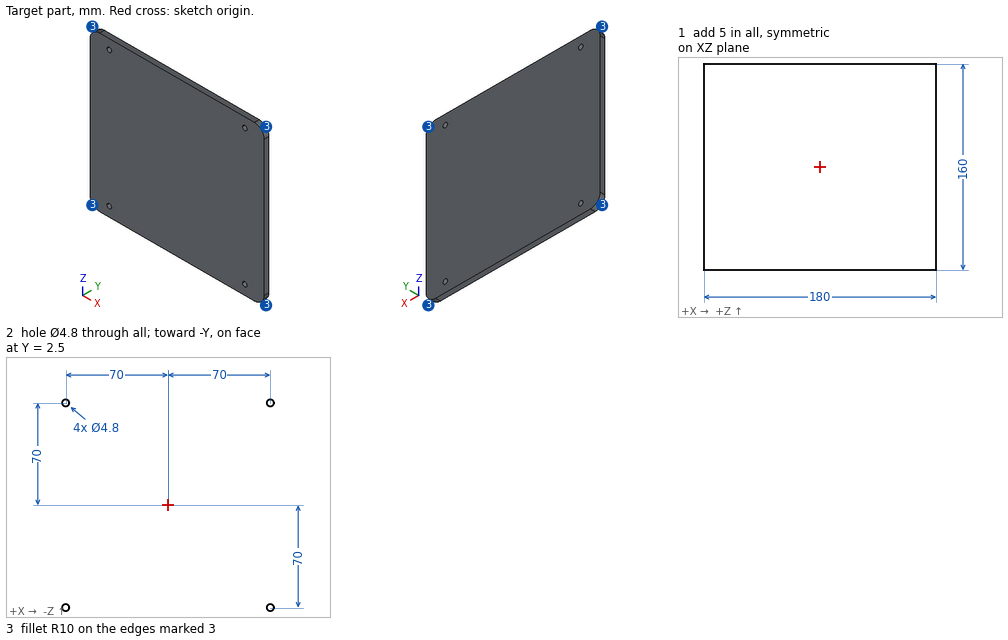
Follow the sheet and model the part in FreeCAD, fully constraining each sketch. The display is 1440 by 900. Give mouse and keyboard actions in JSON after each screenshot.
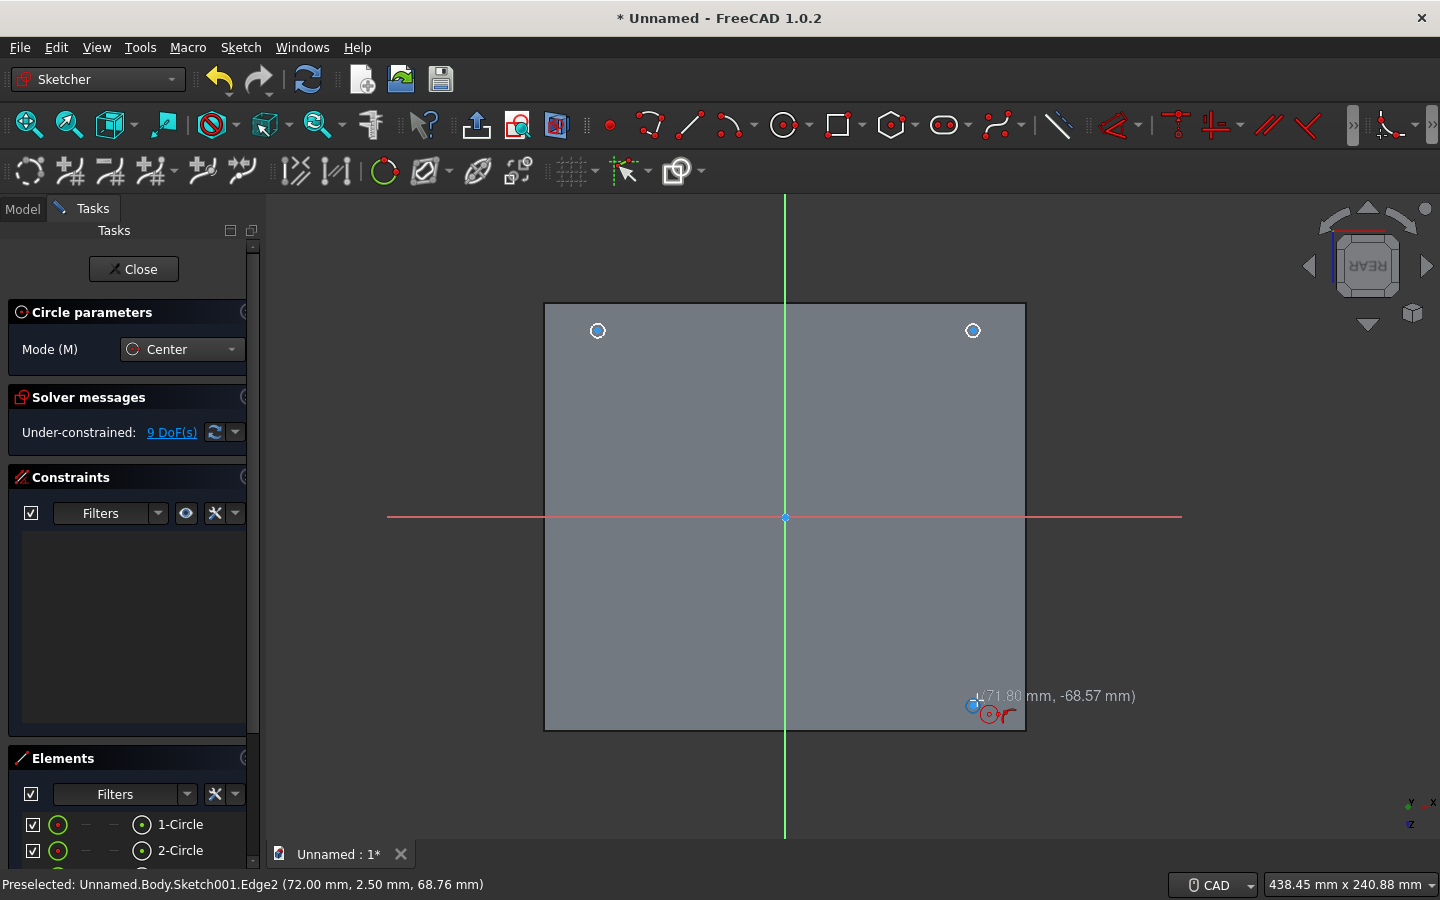
{"action": "scroll", "coordinate": [598, 705], "scroll_direction": "up", "scroll_amount": 7}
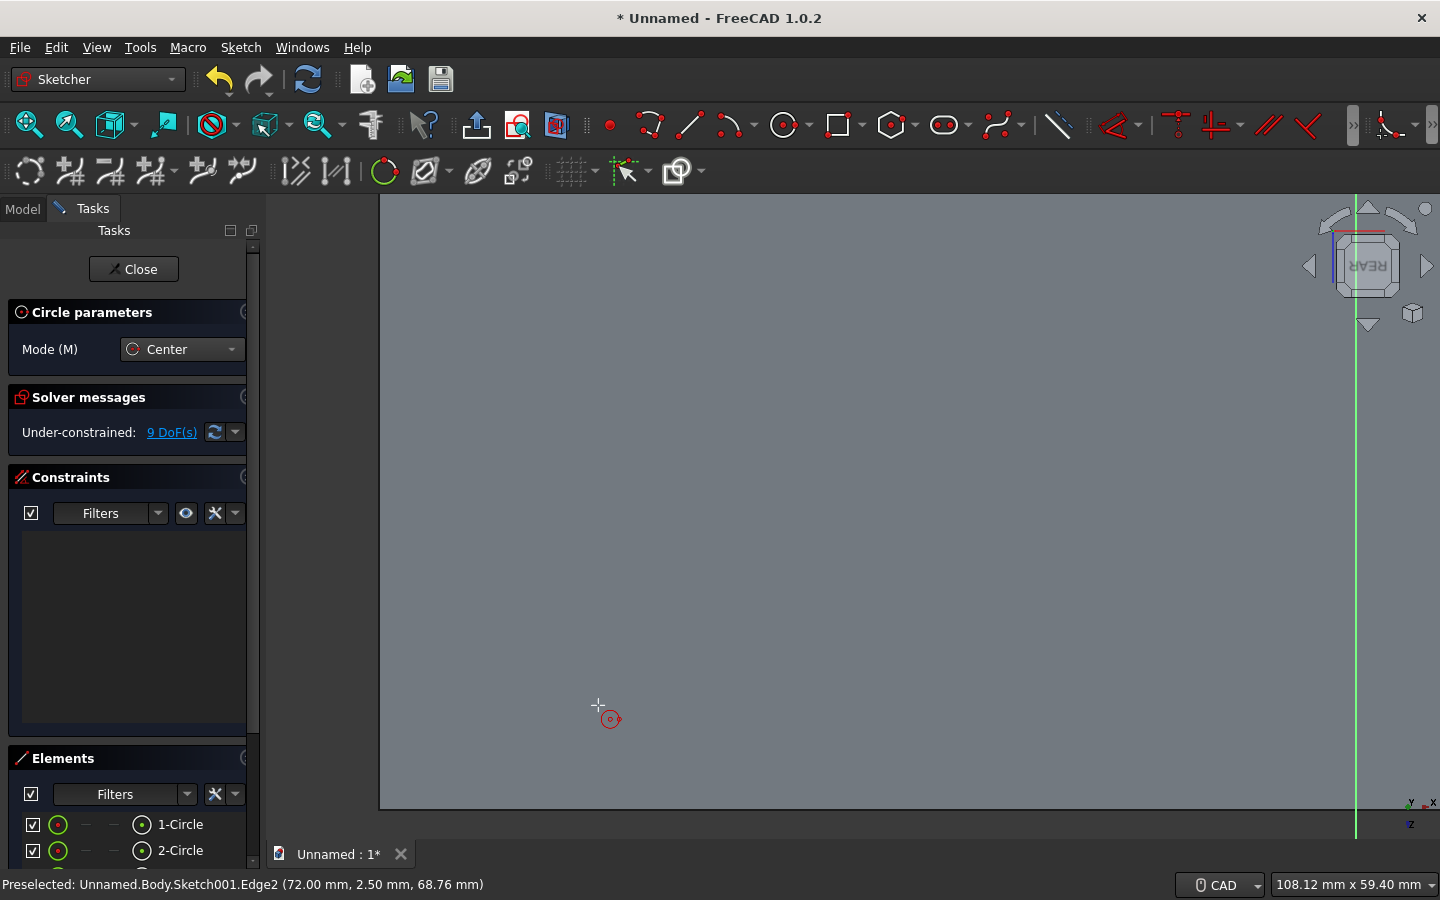
{"action": "scroll", "coordinate": [597, 705], "scroll_direction": "down", "scroll_amount": 7}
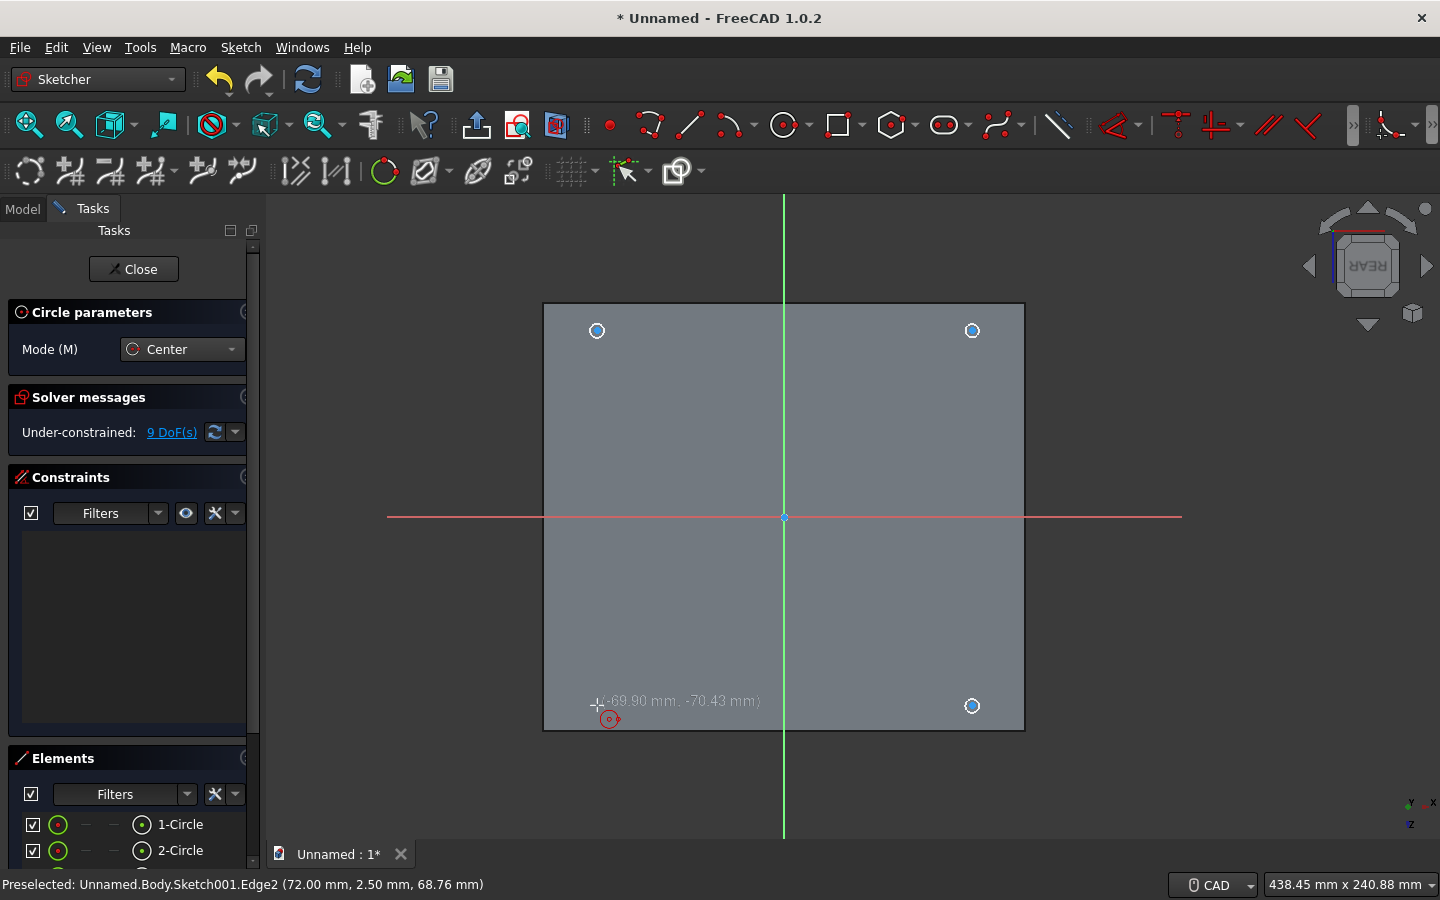
{"action": "left_click", "coordinate": [597, 705]}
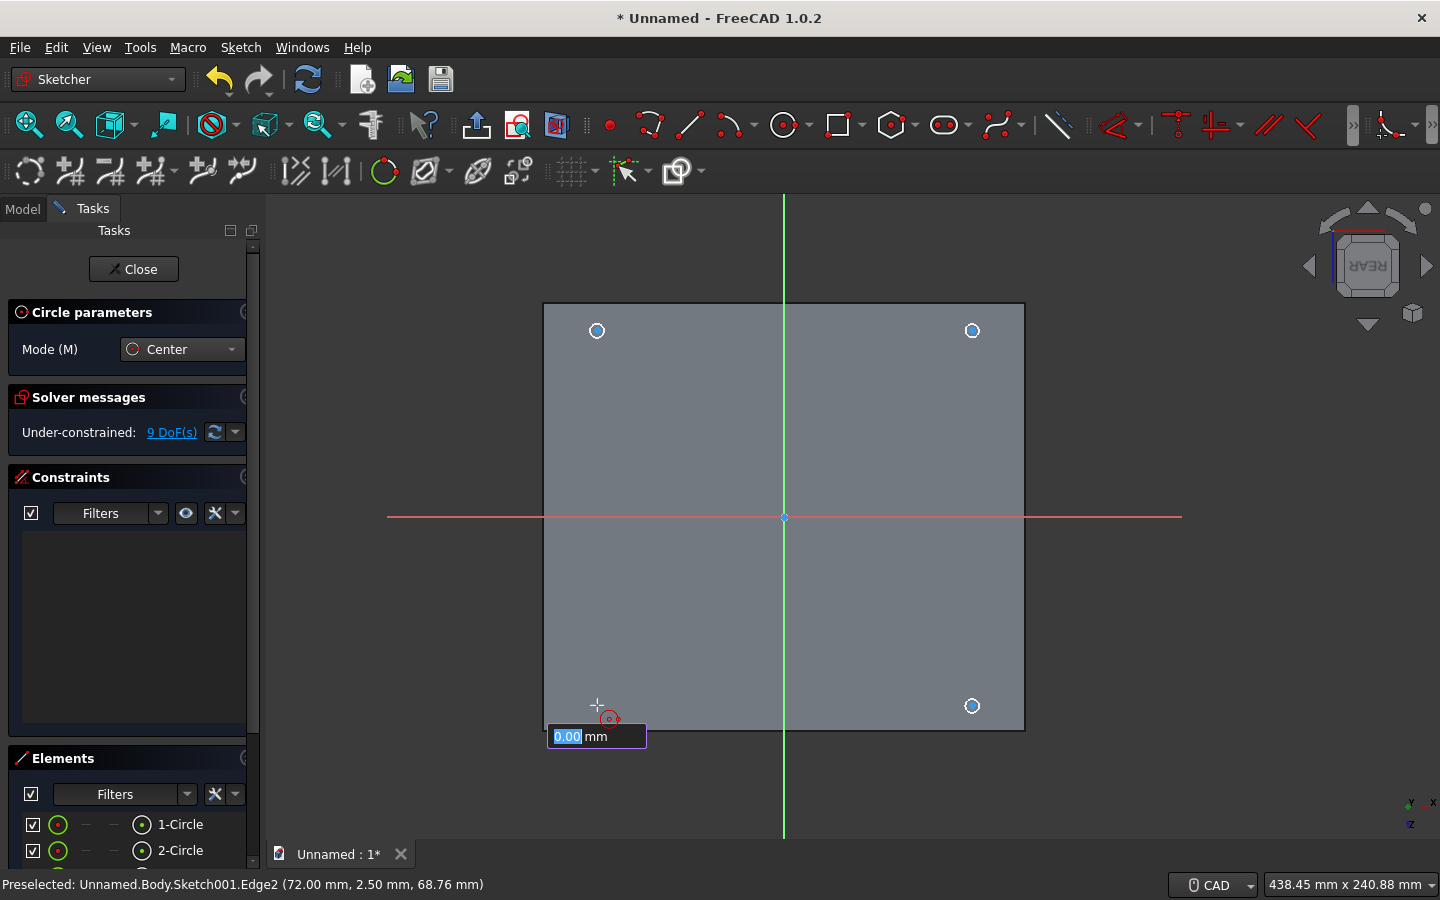
{"action": "scroll", "coordinate": [601, 700], "scroll_direction": "up", "scroll_amount": 5}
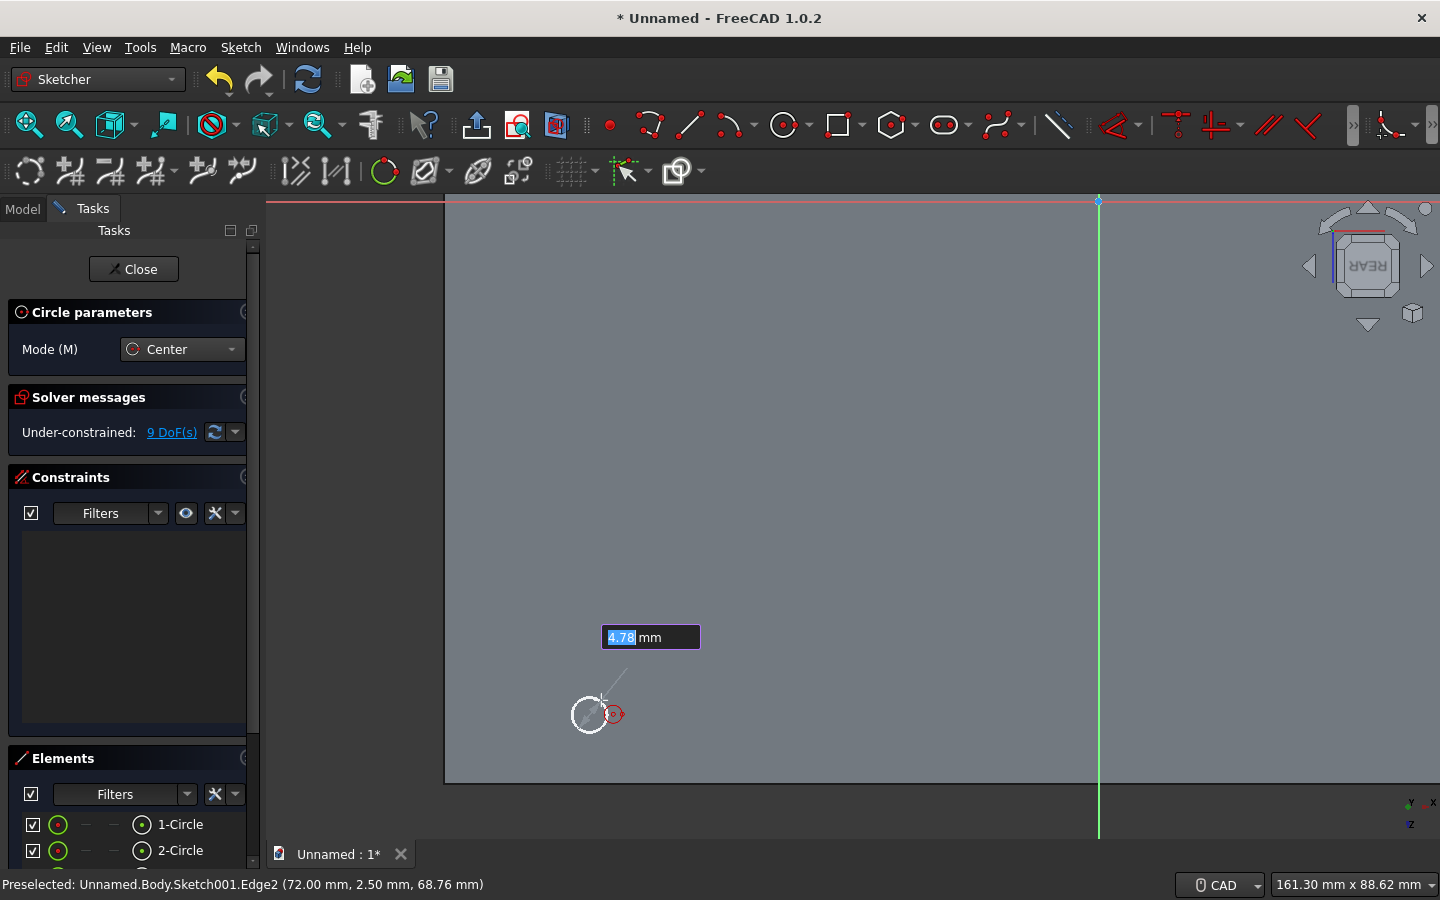
{"action": "left_click", "coordinate": [602, 699]}
{"action": "key", "text": "Escape"}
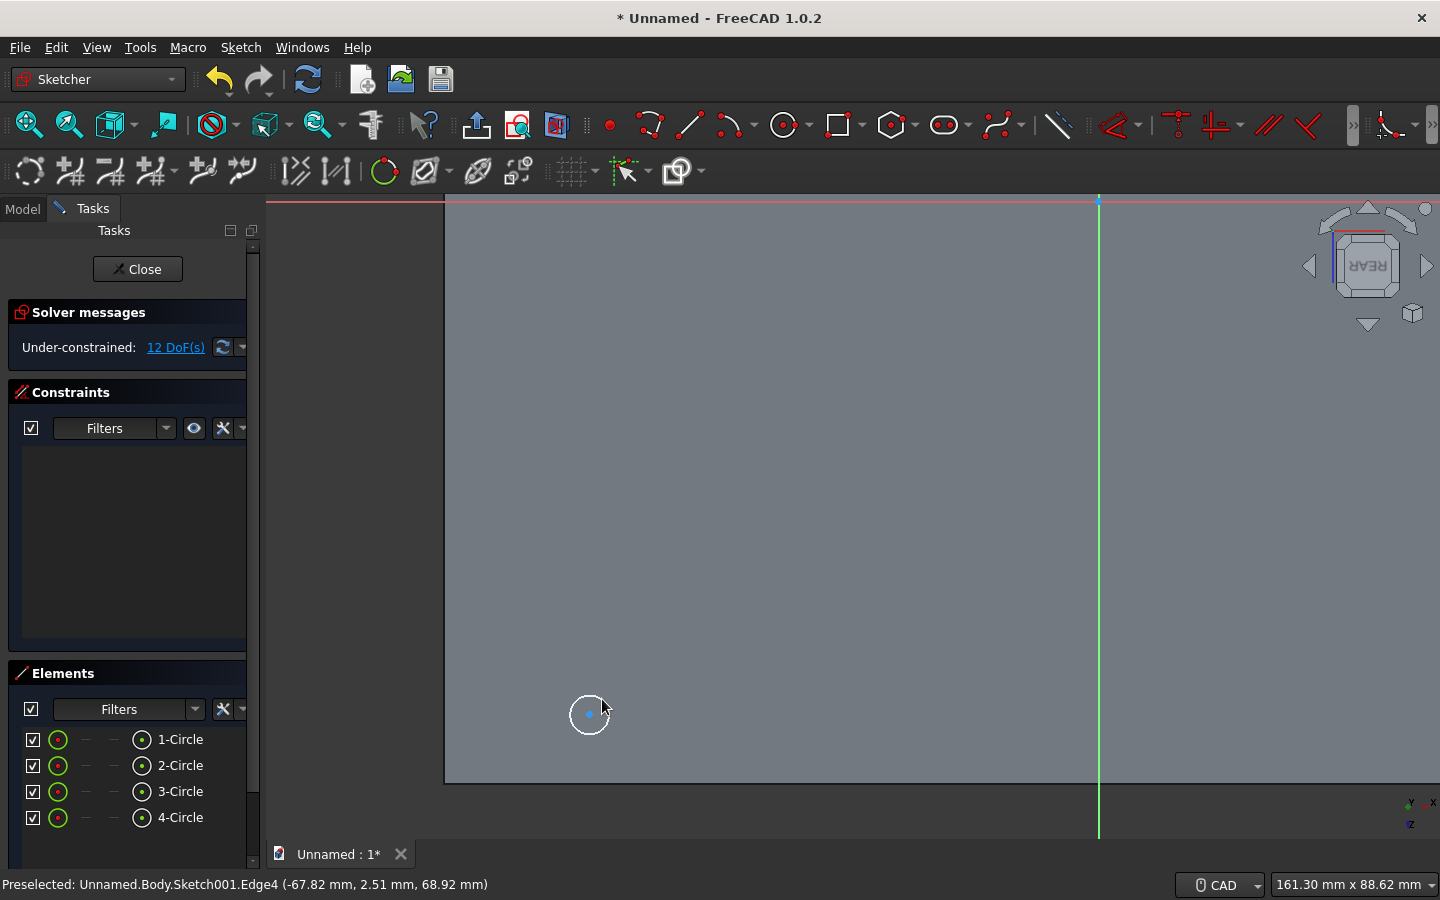
{"action": "scroll", "coordinate": [601, 700], "scroll_direction": "down", "scroll_amount": 5}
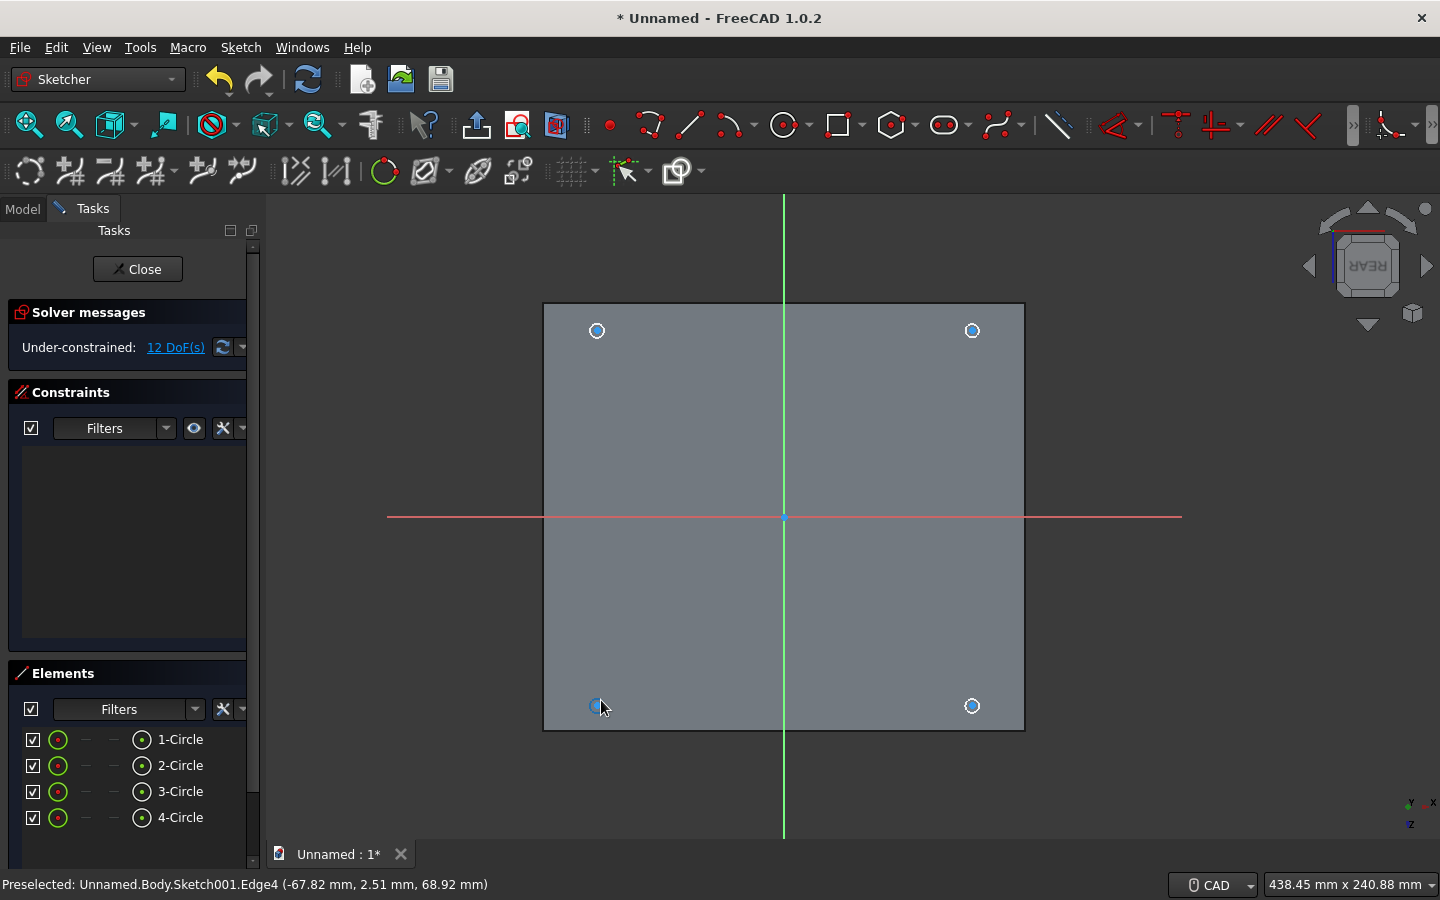
{"action": "scroll", "coordinate": [602, 326], "scroll_direction": "up", "scroll_amount": 4}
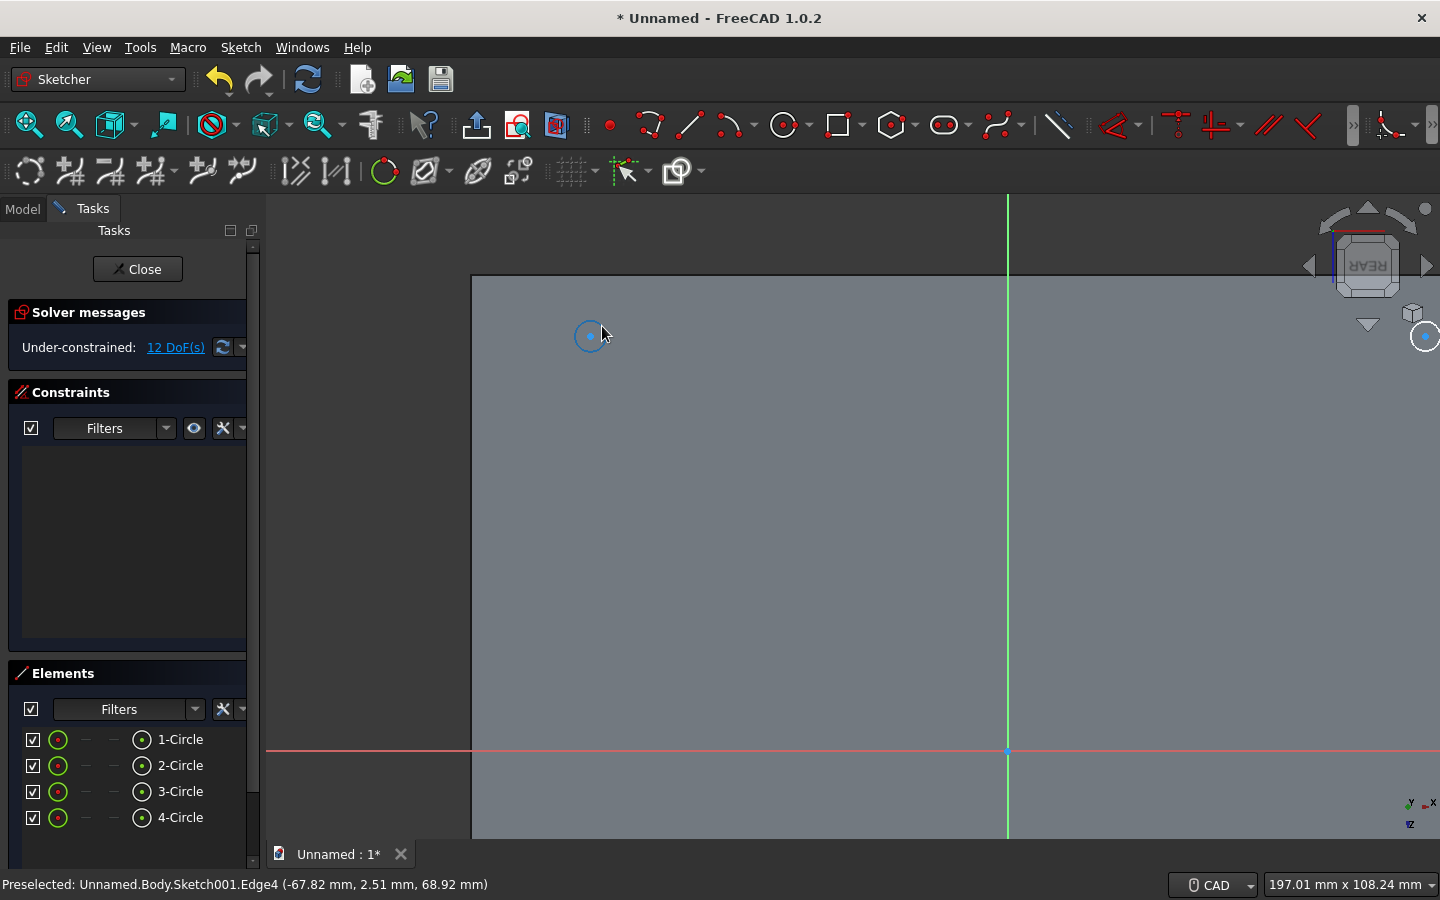
{"action": "left_click", "coordinate": [601, 325]}